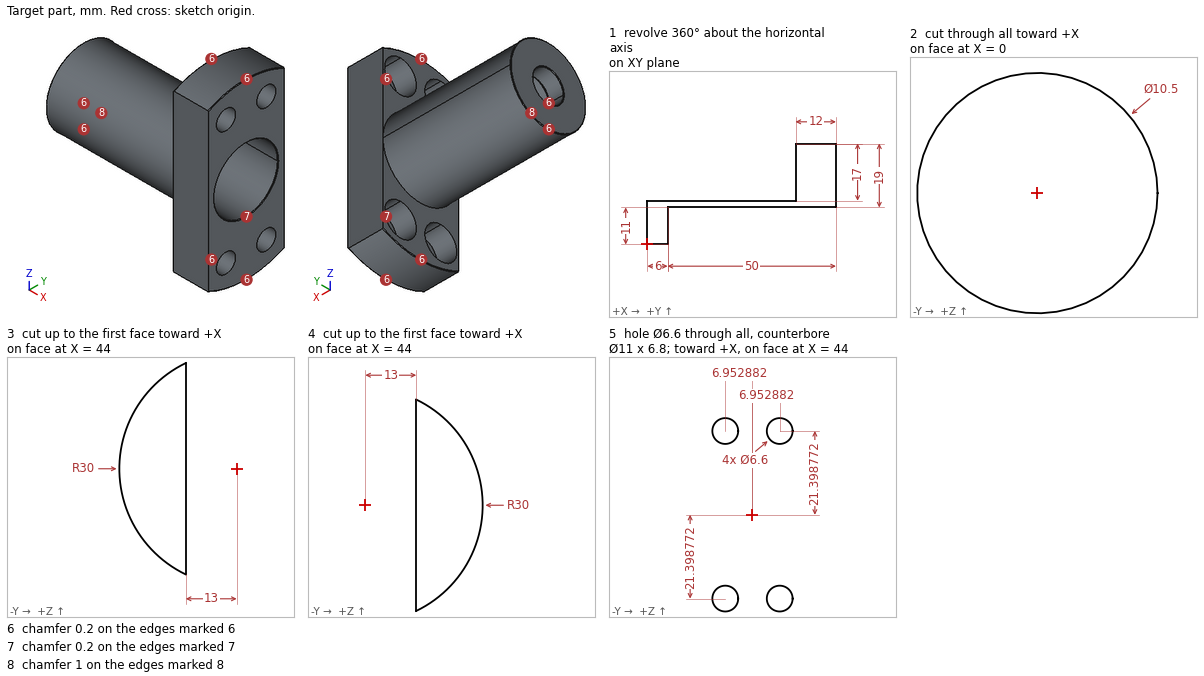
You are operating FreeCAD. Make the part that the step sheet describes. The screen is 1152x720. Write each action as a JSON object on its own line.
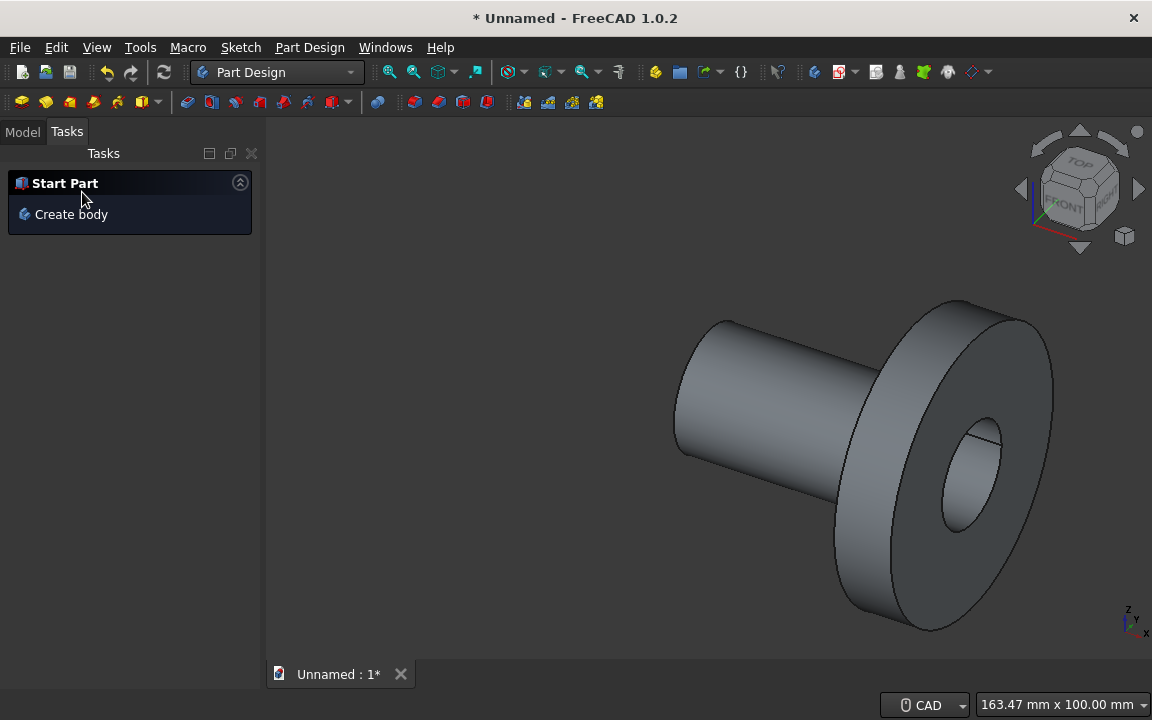
{"action": "left_click", "coordinate": [390, 72]}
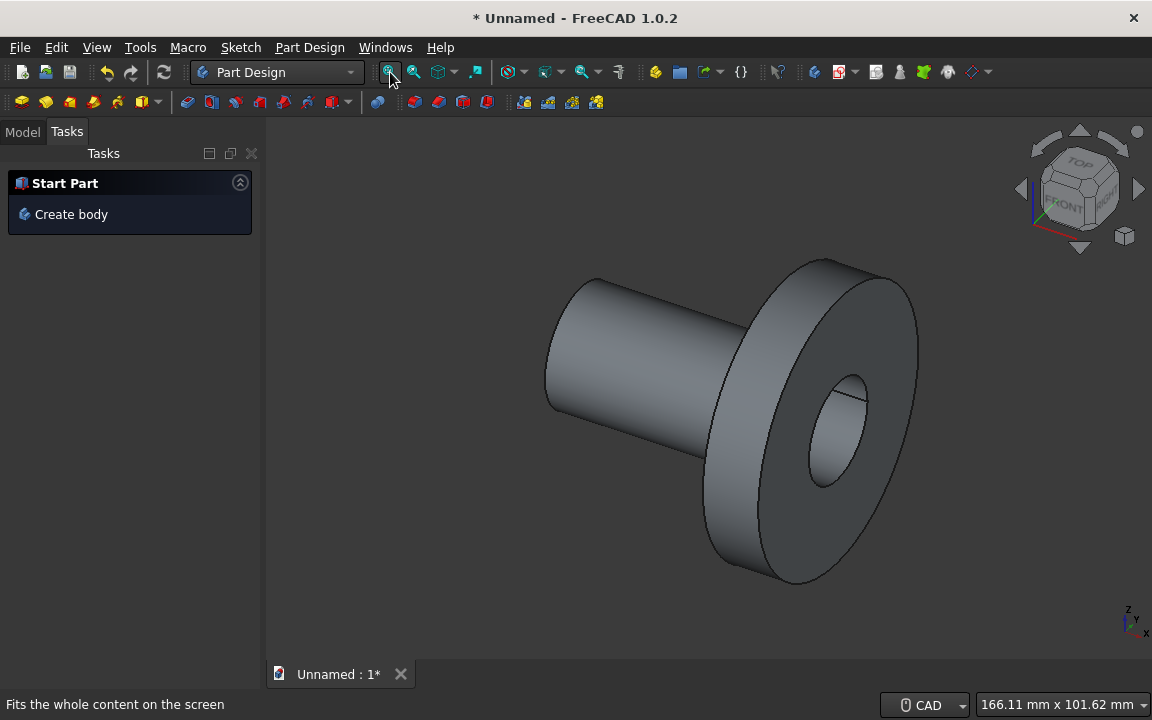
{"action": "key", "text": "6"}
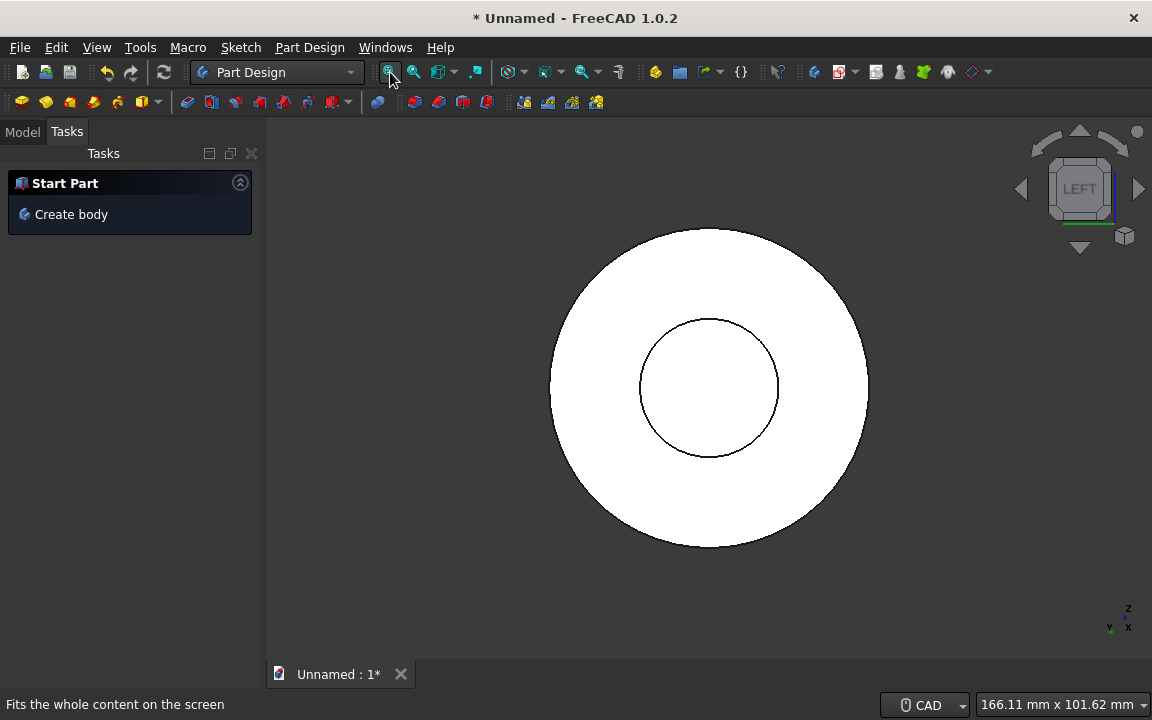
{"action": "left_click", "coordinate": [709, 387]}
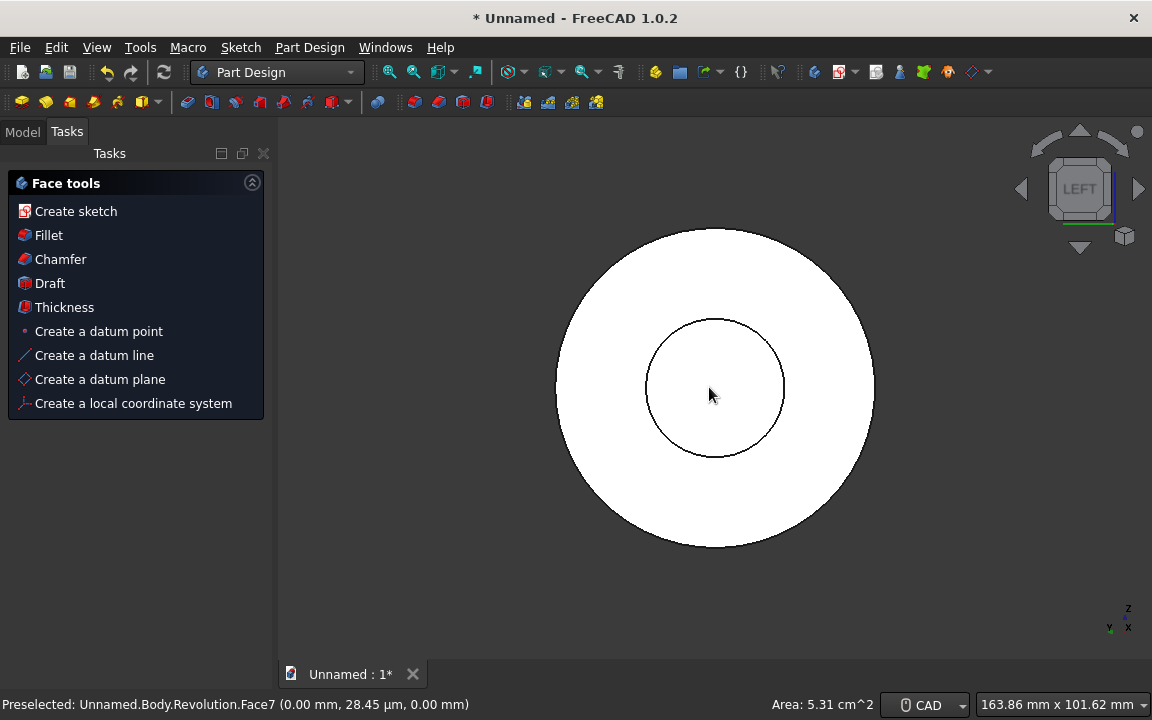
{"action": "left_click", "coordinate": [840, 72]}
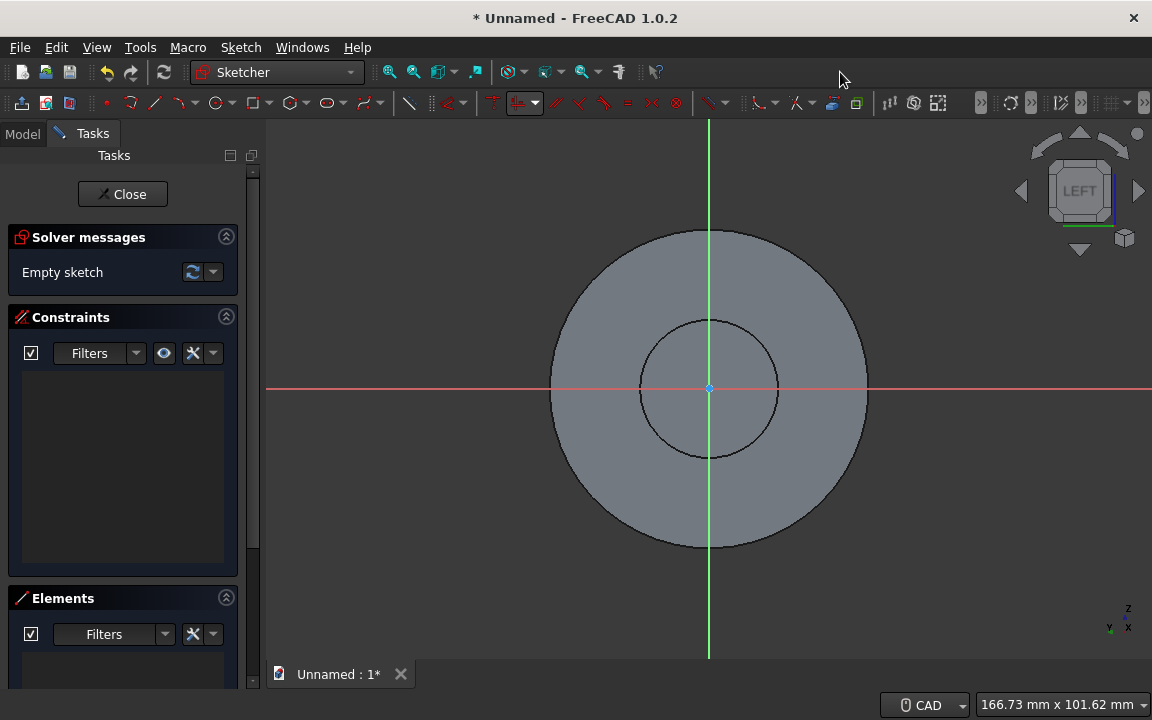
{"action": "scroll", "coordinate": [723, 389], "scroll_direction": "up", "scroll_amount": 9}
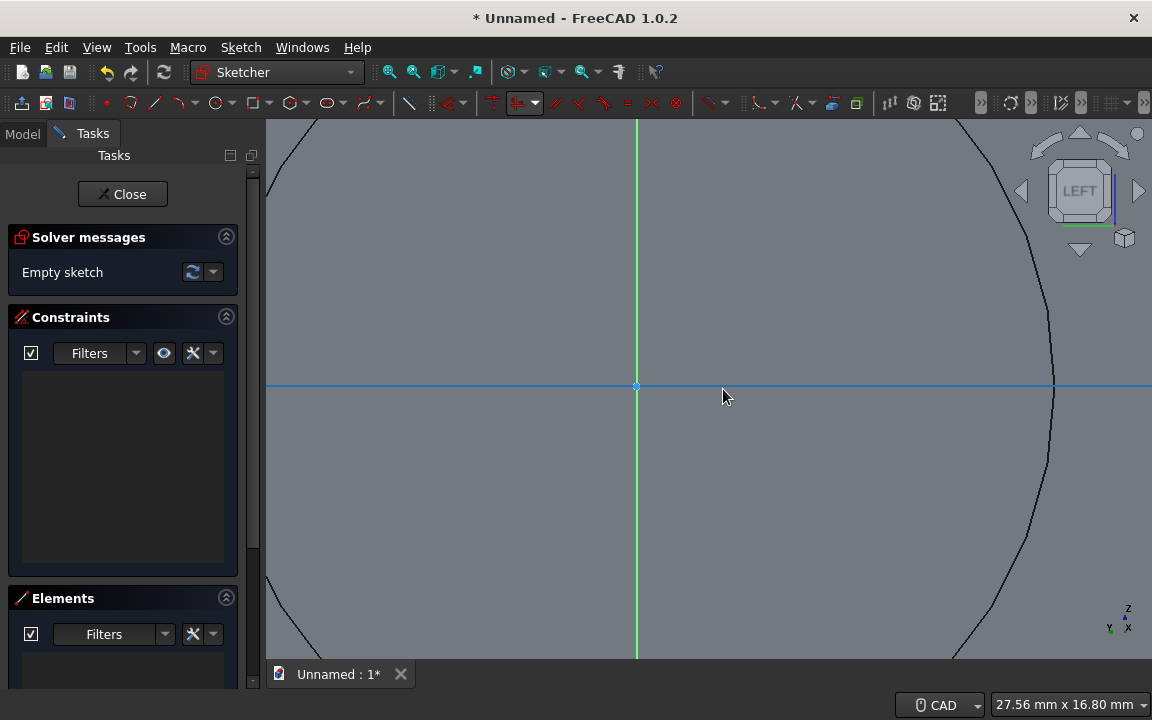
{"action": "left_click", "coordinate": [216, 104]}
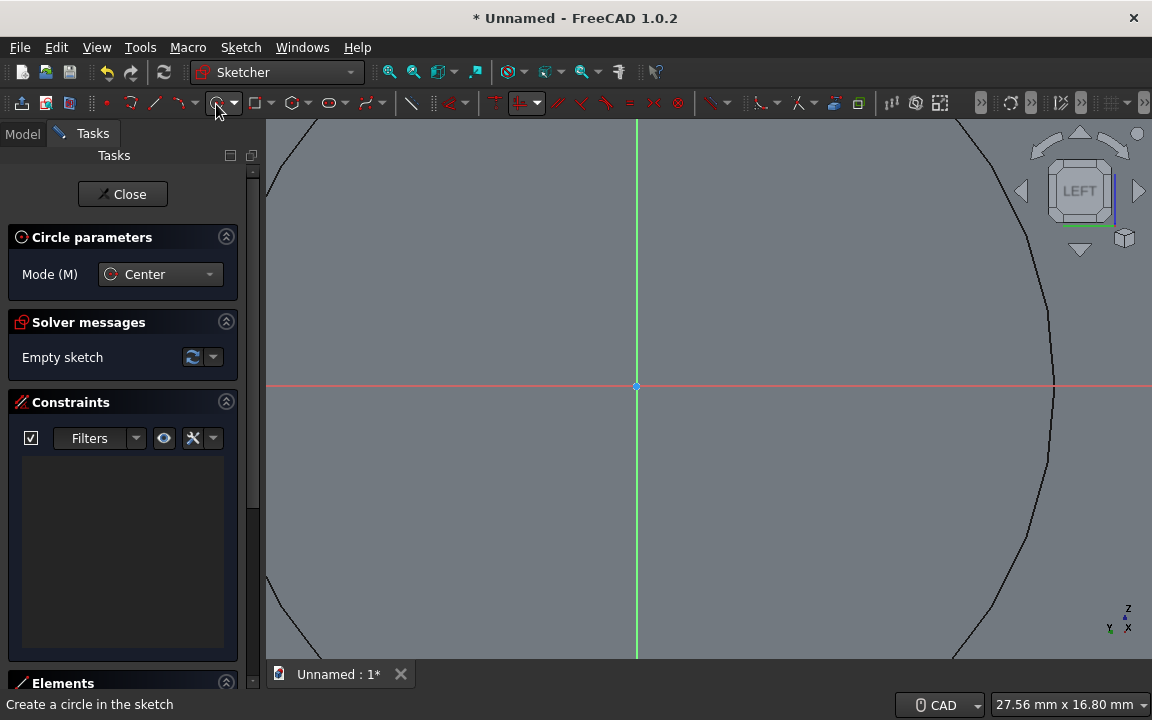
{"action": "left_click", "coordinate": [637, 386]}
{"action": "mouse_move", "coordinate": [756, 267]}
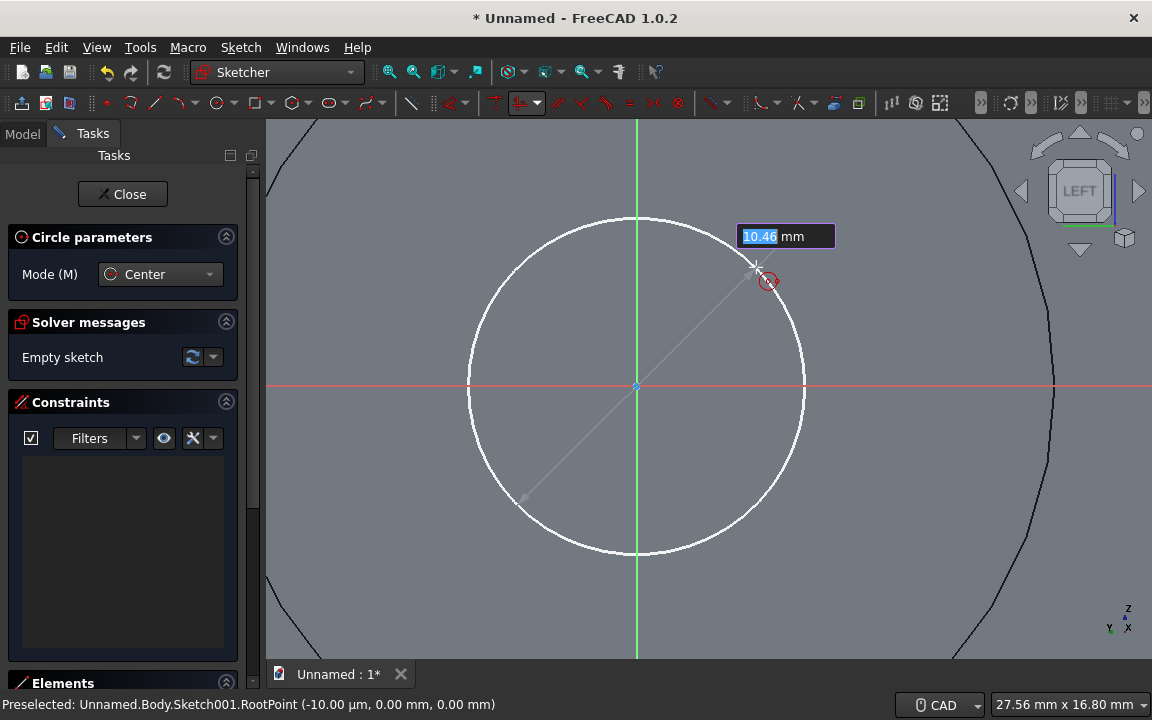
{"action": "type", "text": "10.5"}
{"action": "key", "text": "Return"}
{"action": "key", "text": "Escape"}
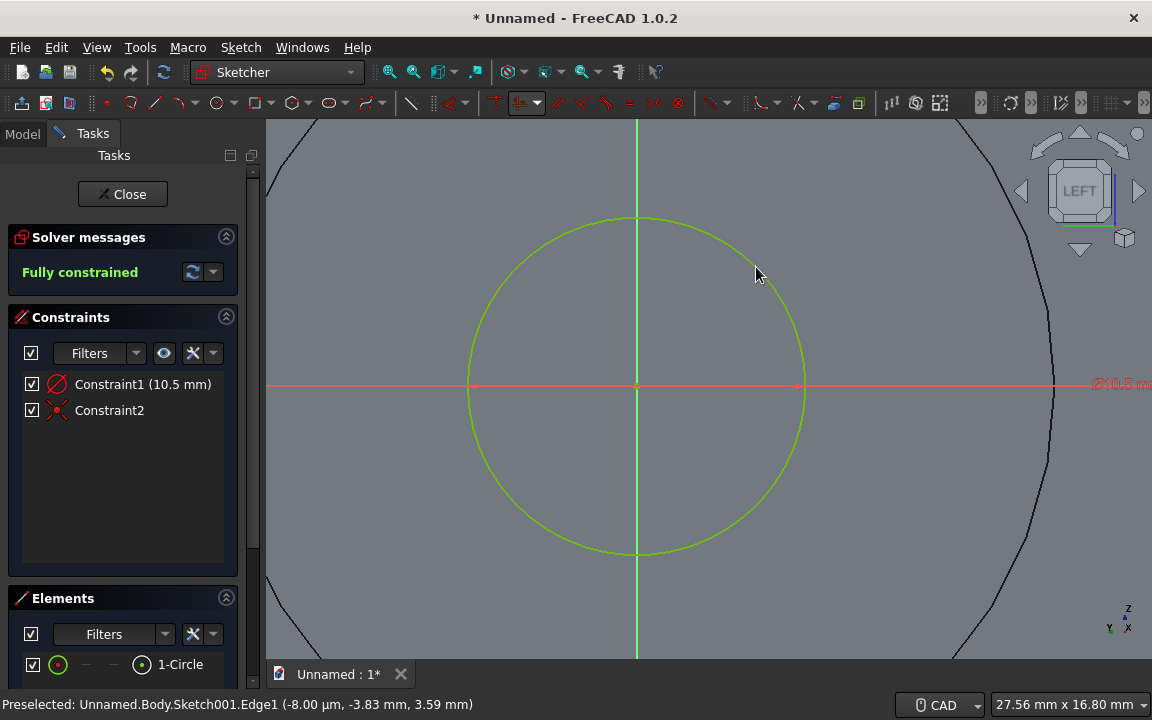
{"action": "left_click", "coordinate": [123, 194]}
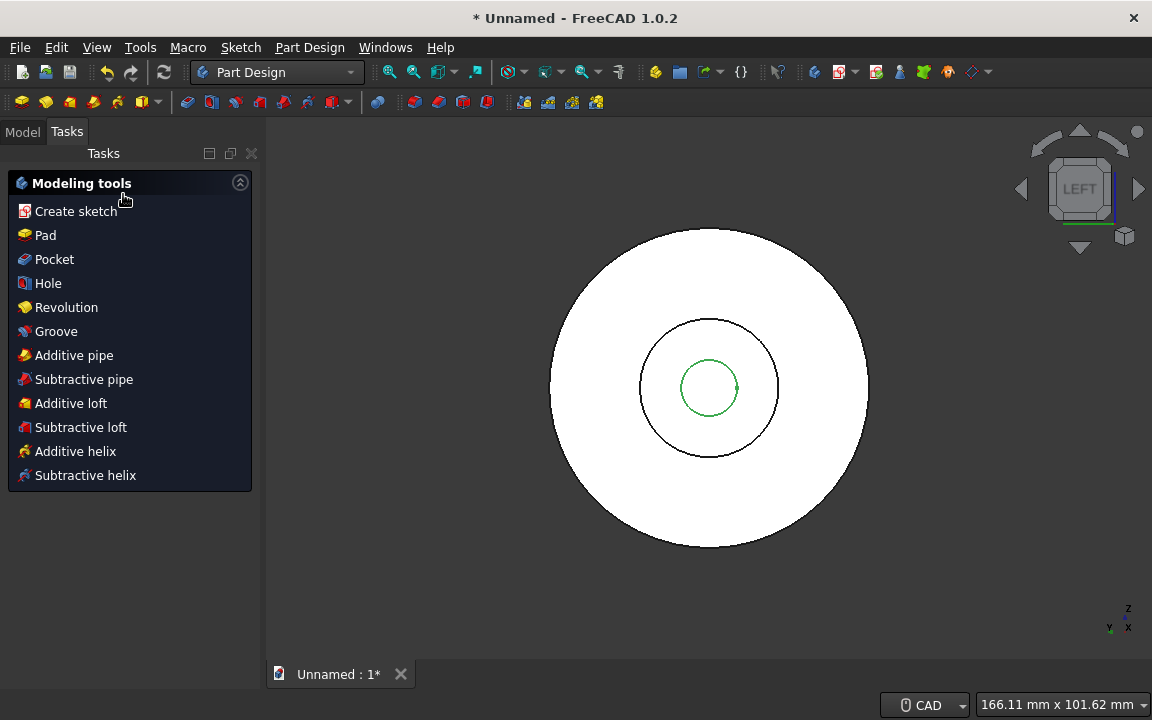
{"action": "left_click", "coordinate": [188, 102]}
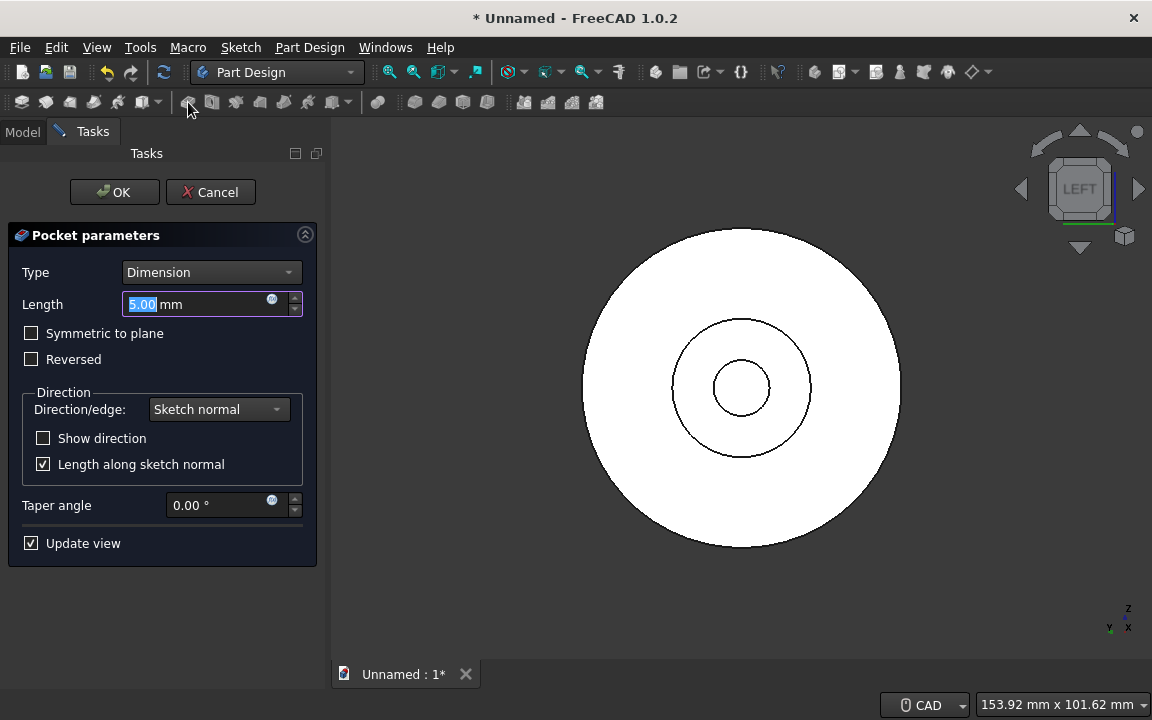
{"action": "left_click", "coordinate": [212, 272]}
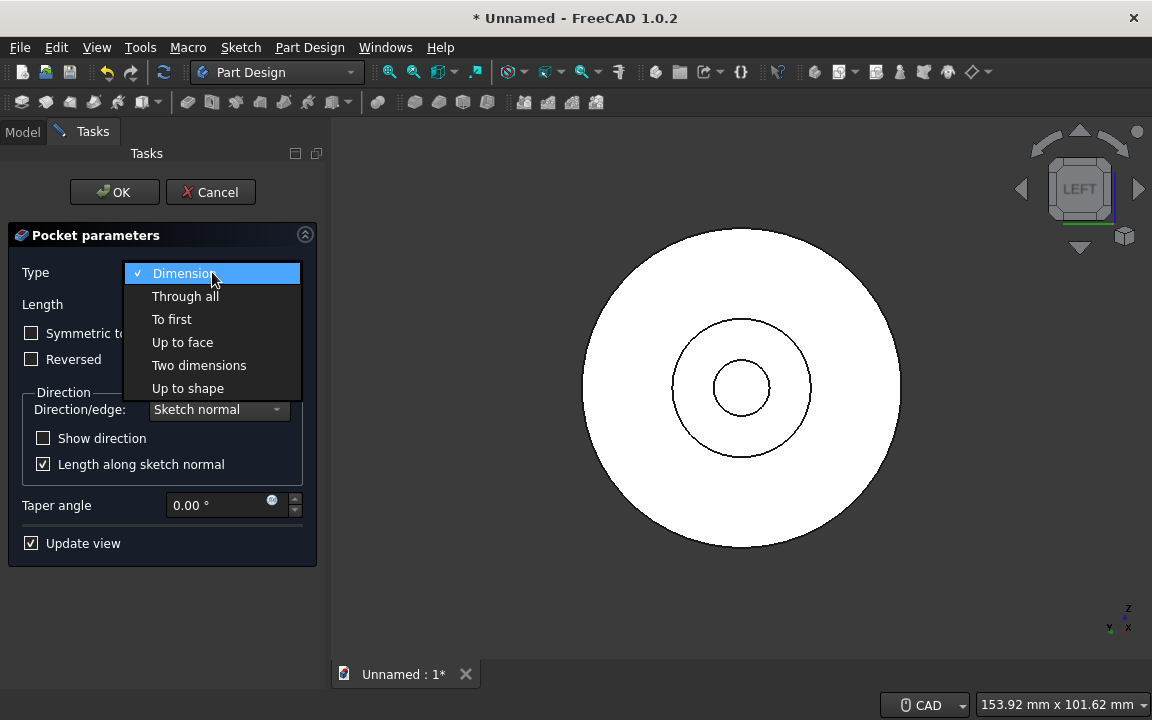
{"action": "left_click", "coordinate": [212, 296]}